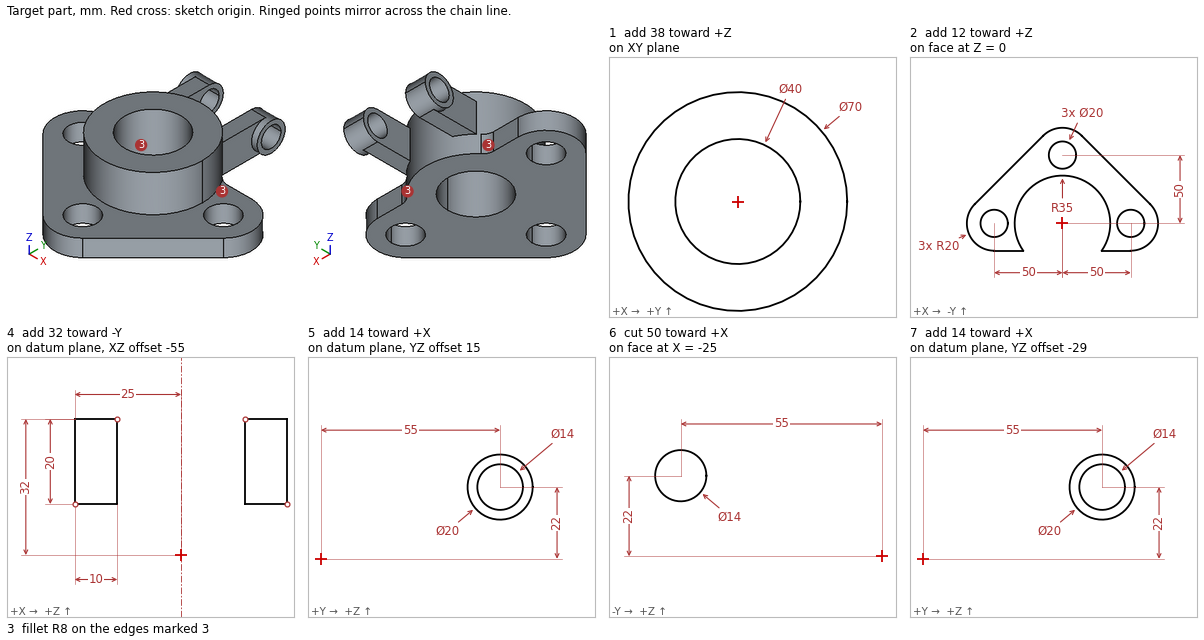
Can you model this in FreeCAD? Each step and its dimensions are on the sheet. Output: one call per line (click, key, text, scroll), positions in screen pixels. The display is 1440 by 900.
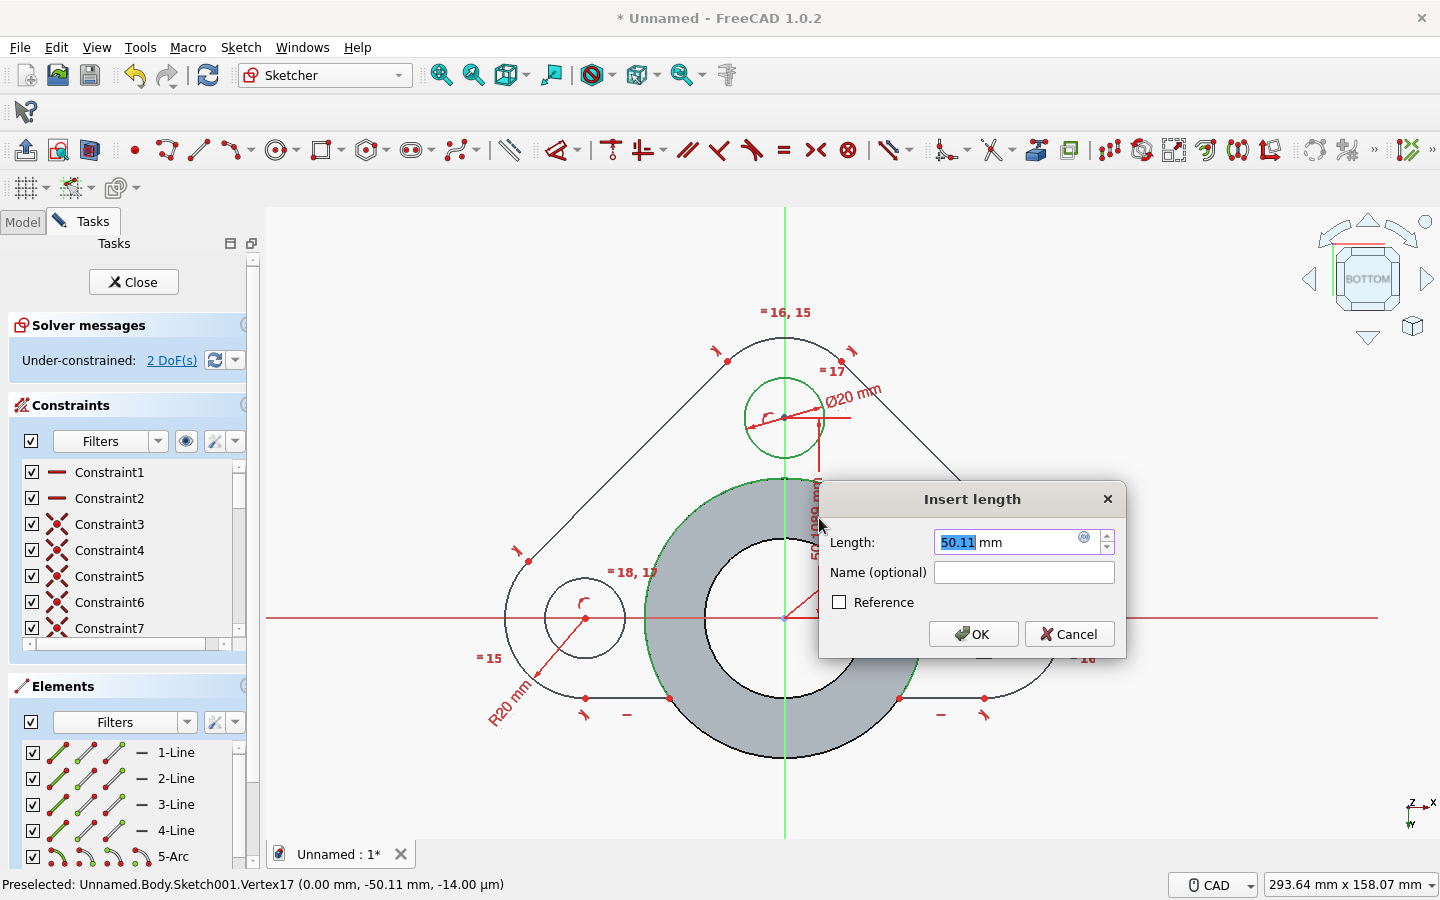
text(50)
key(Return)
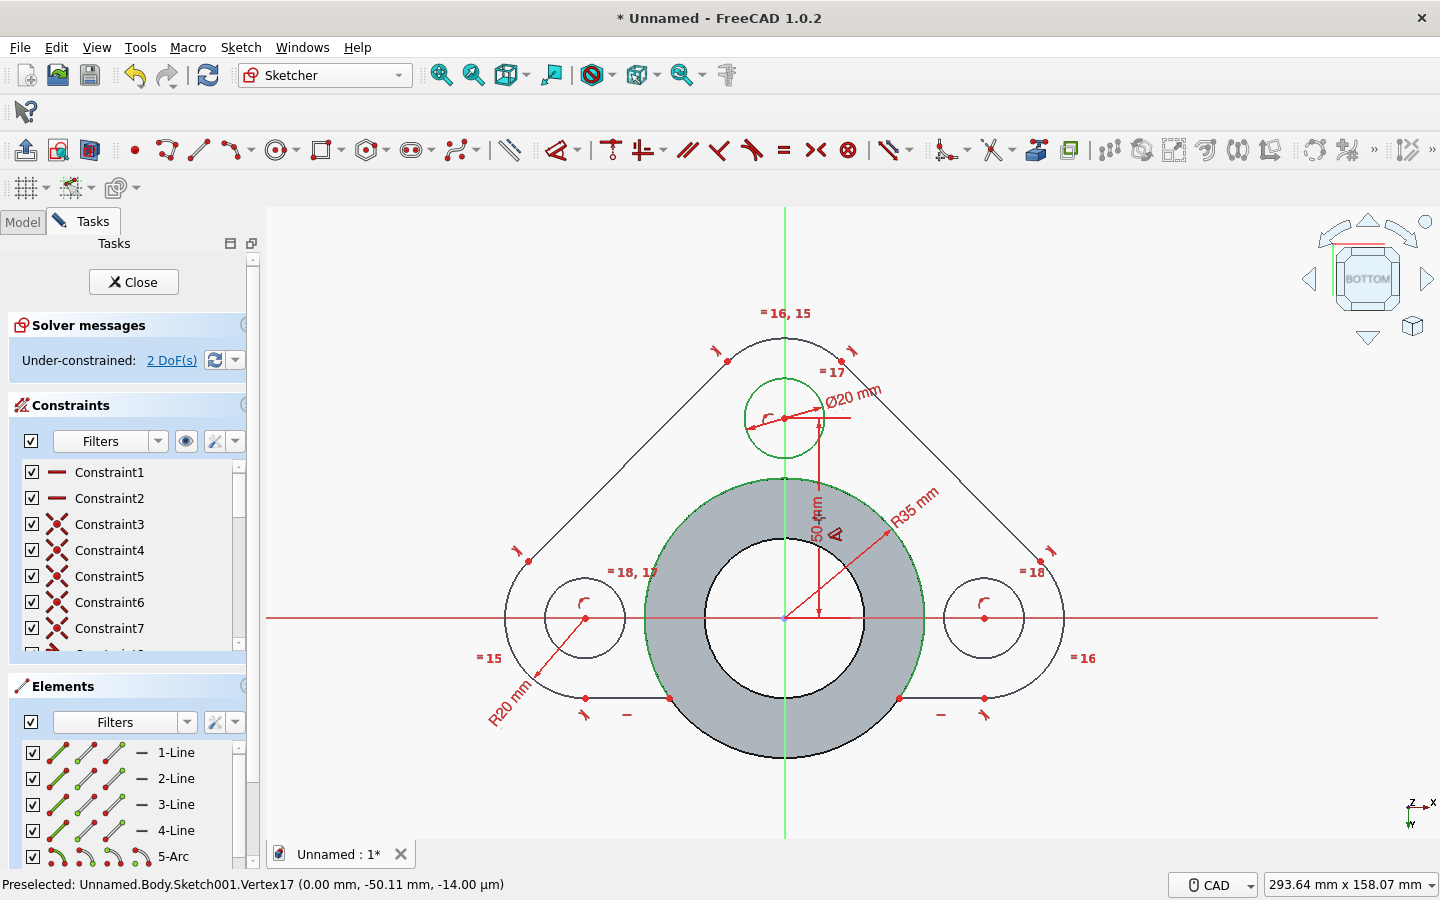
click(585, 618)
click(685, 652)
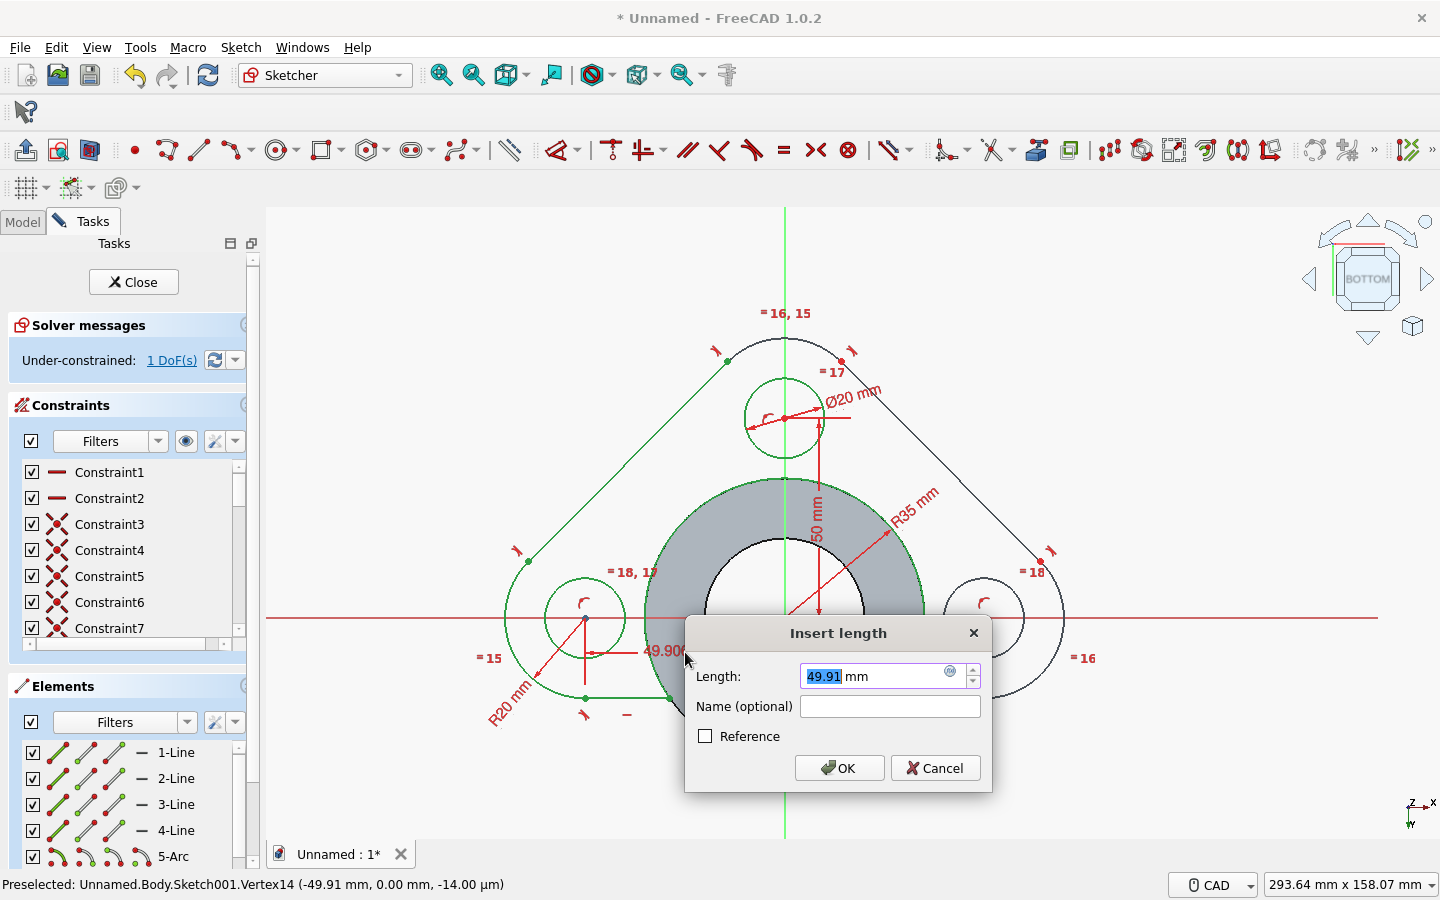
text(50)
key(Return)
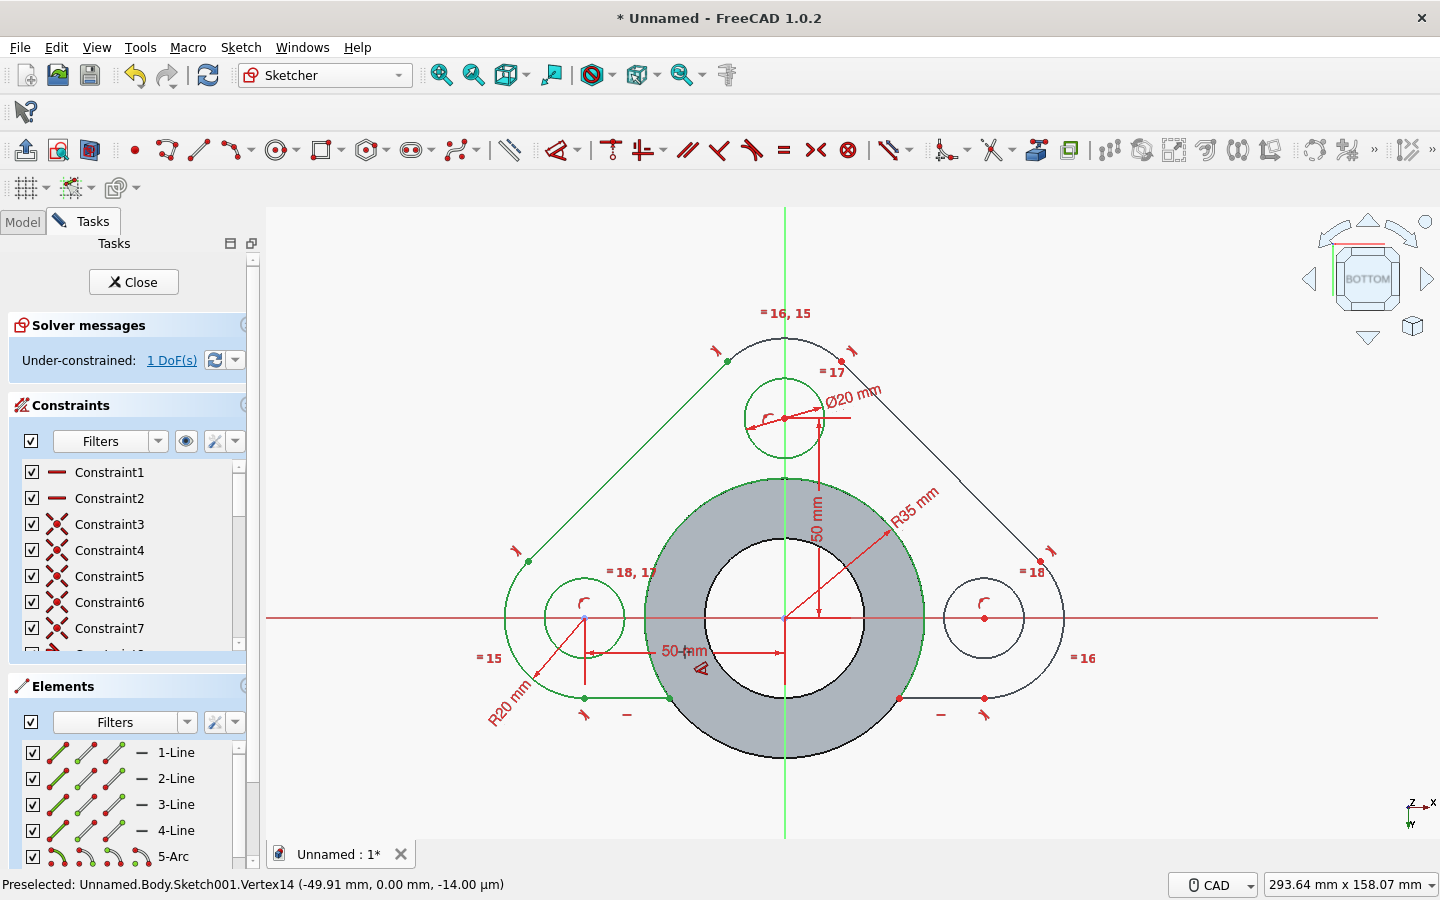
click(984, 618)
click(884, 652)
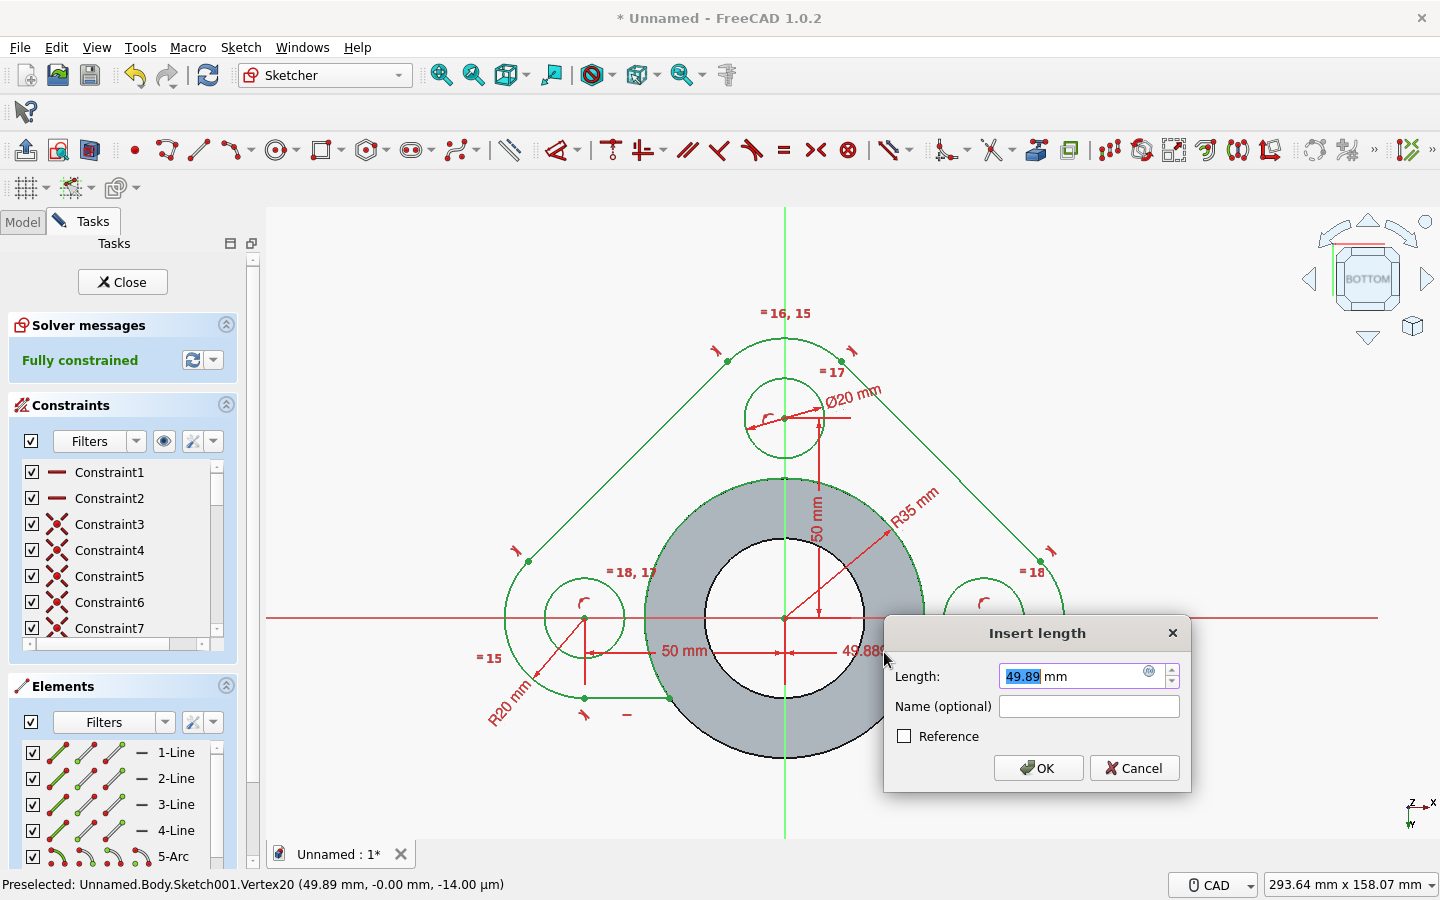
text(50)
key(Return)
key(Escape)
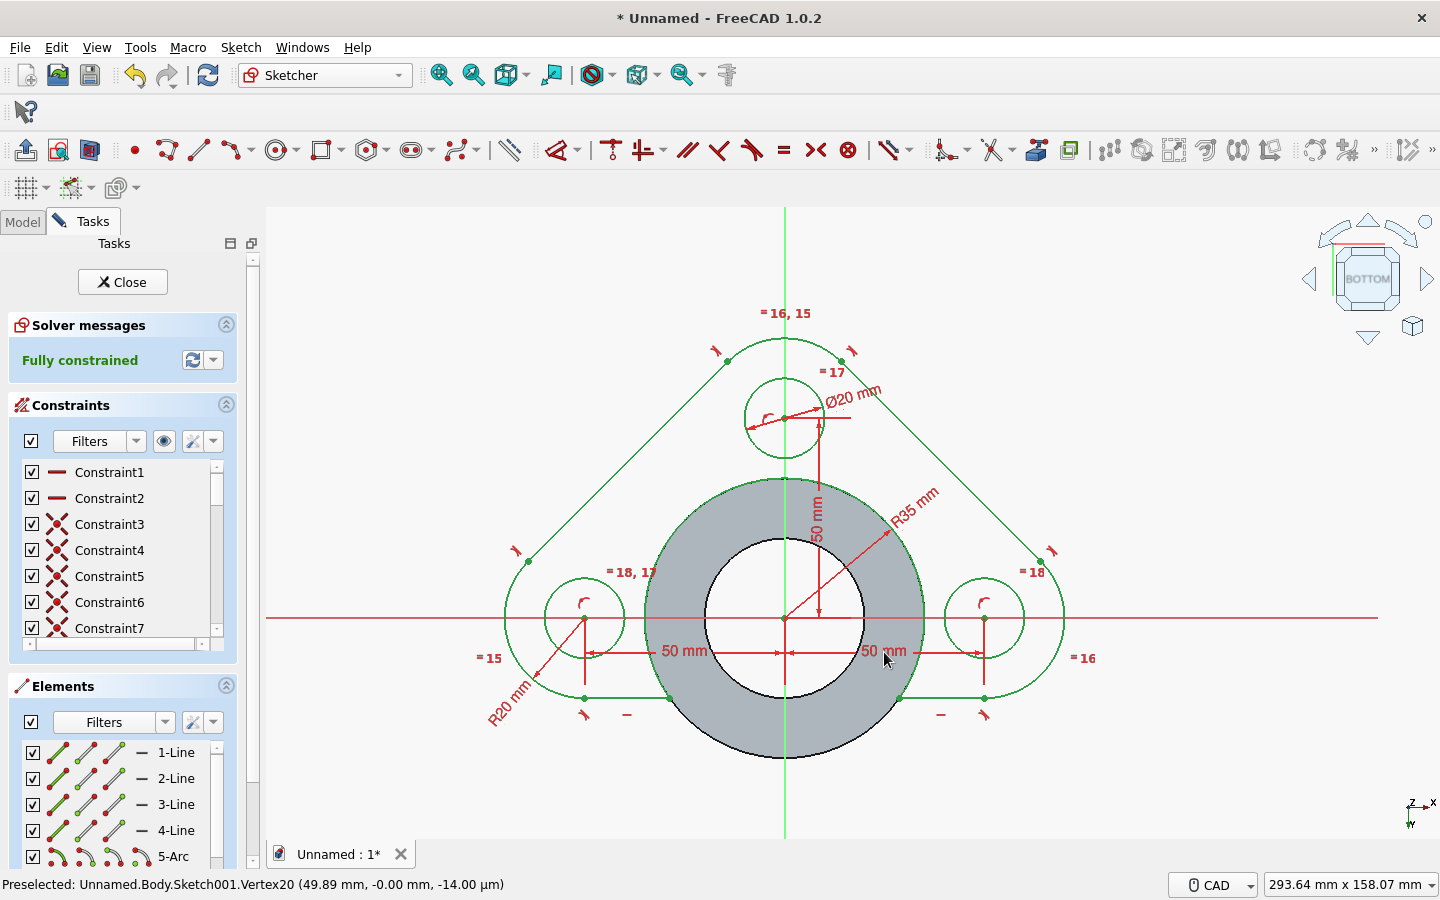
click(123, 282)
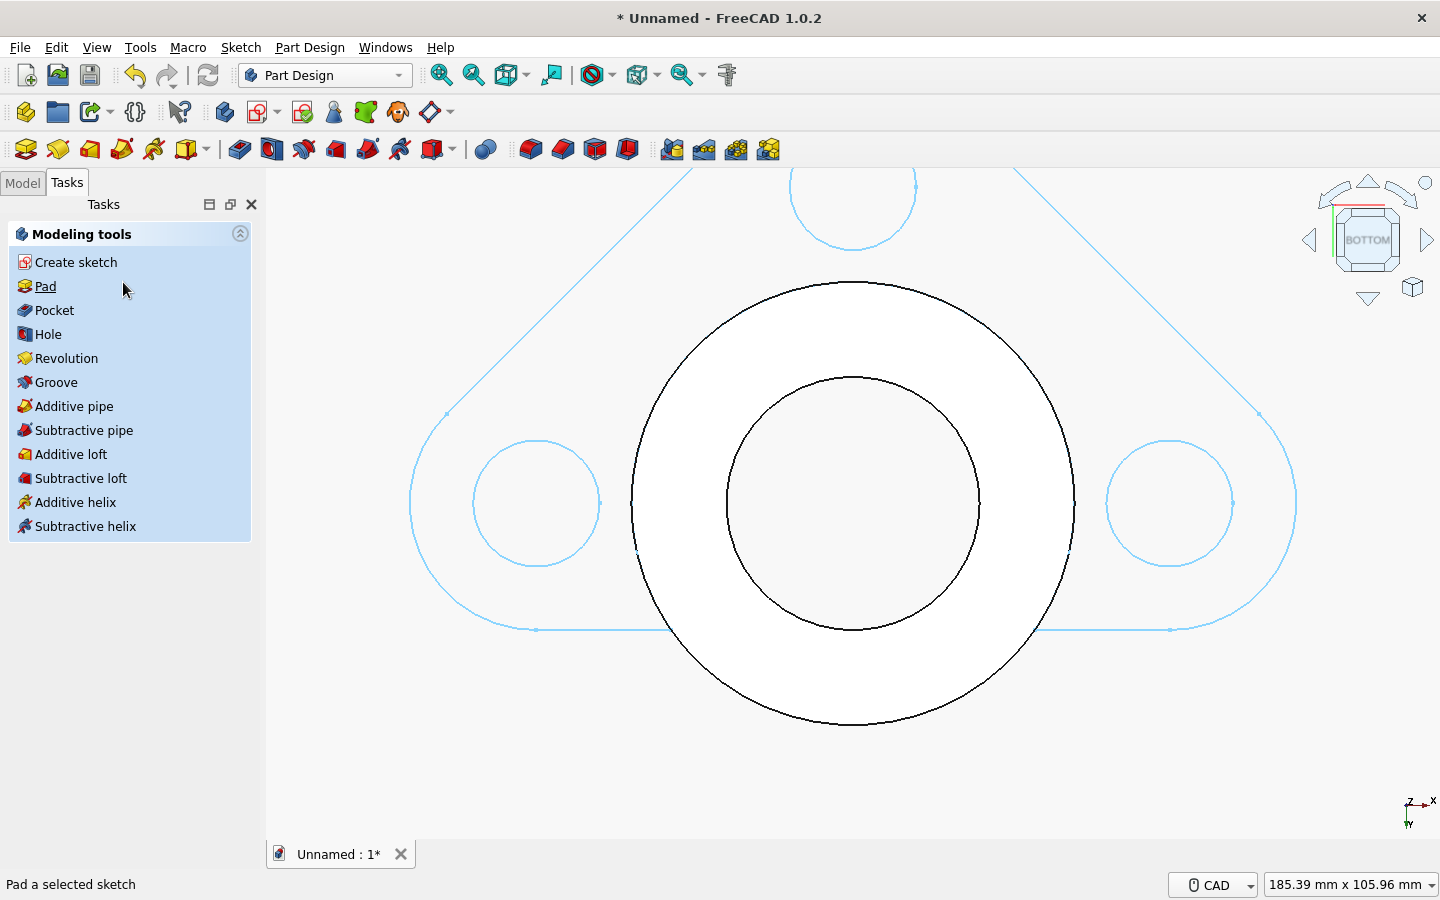
click(26, 150)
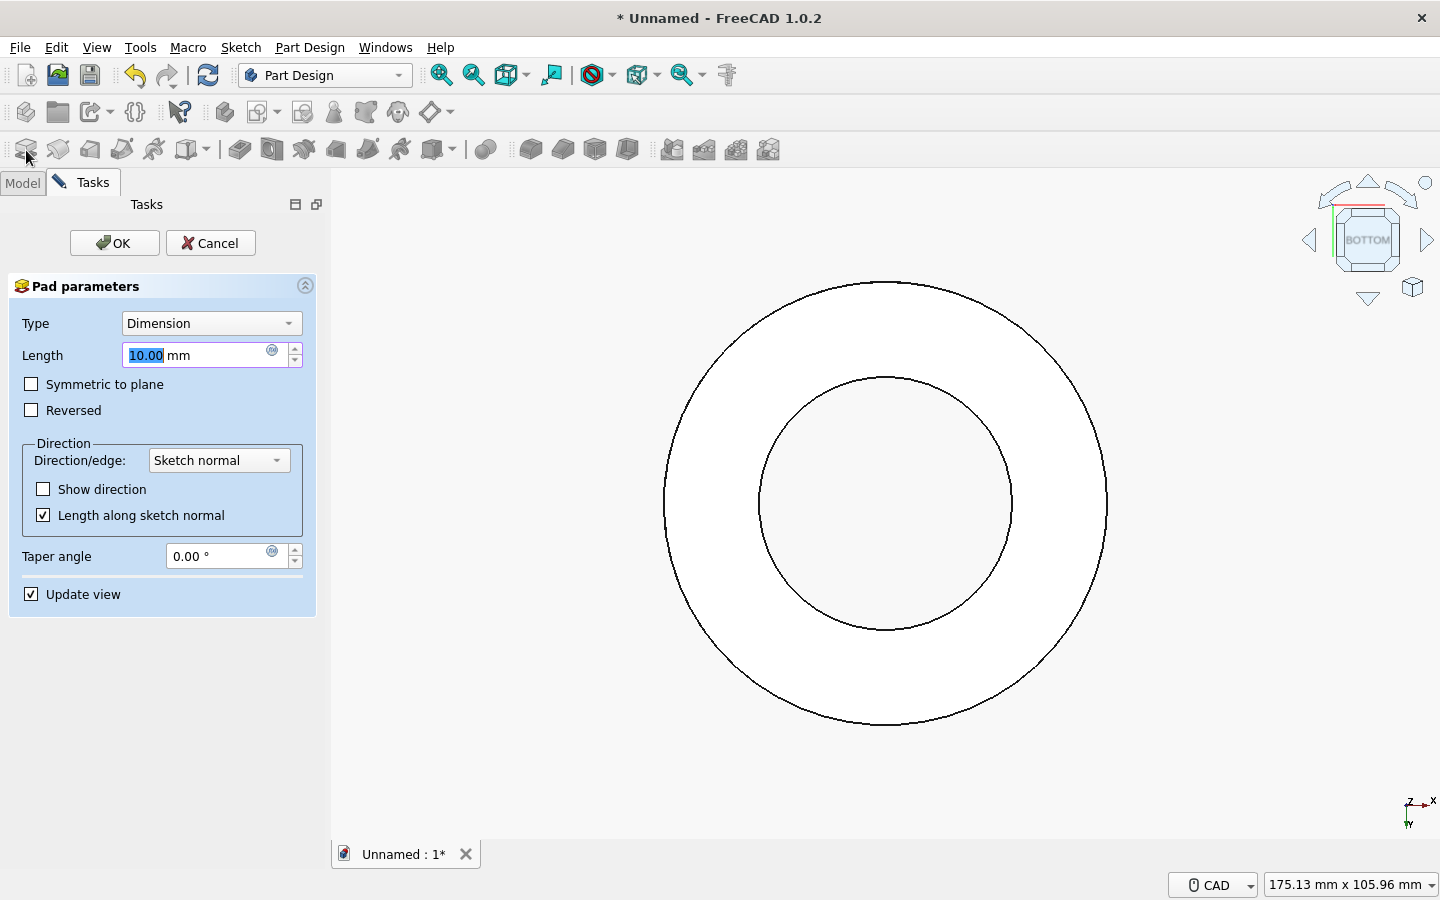
text(12)
key(Tab)